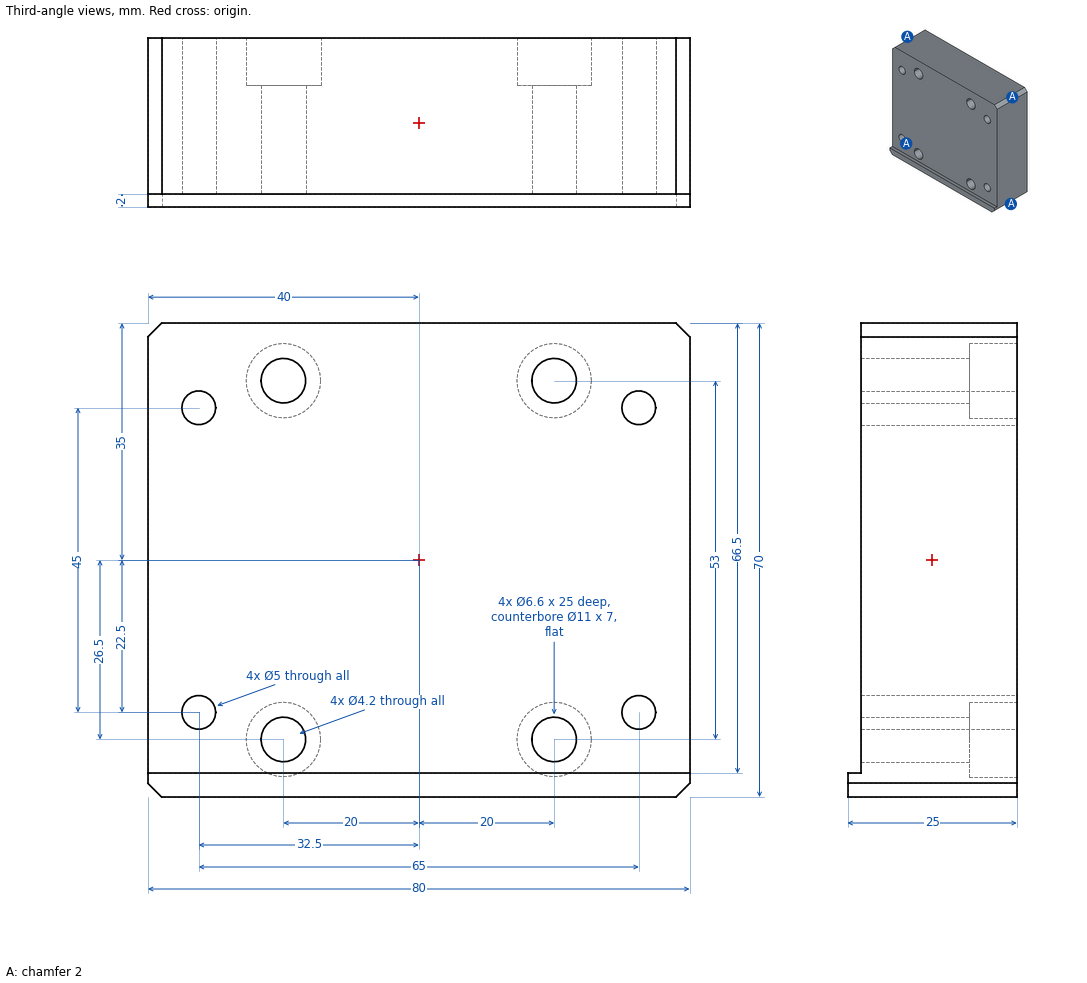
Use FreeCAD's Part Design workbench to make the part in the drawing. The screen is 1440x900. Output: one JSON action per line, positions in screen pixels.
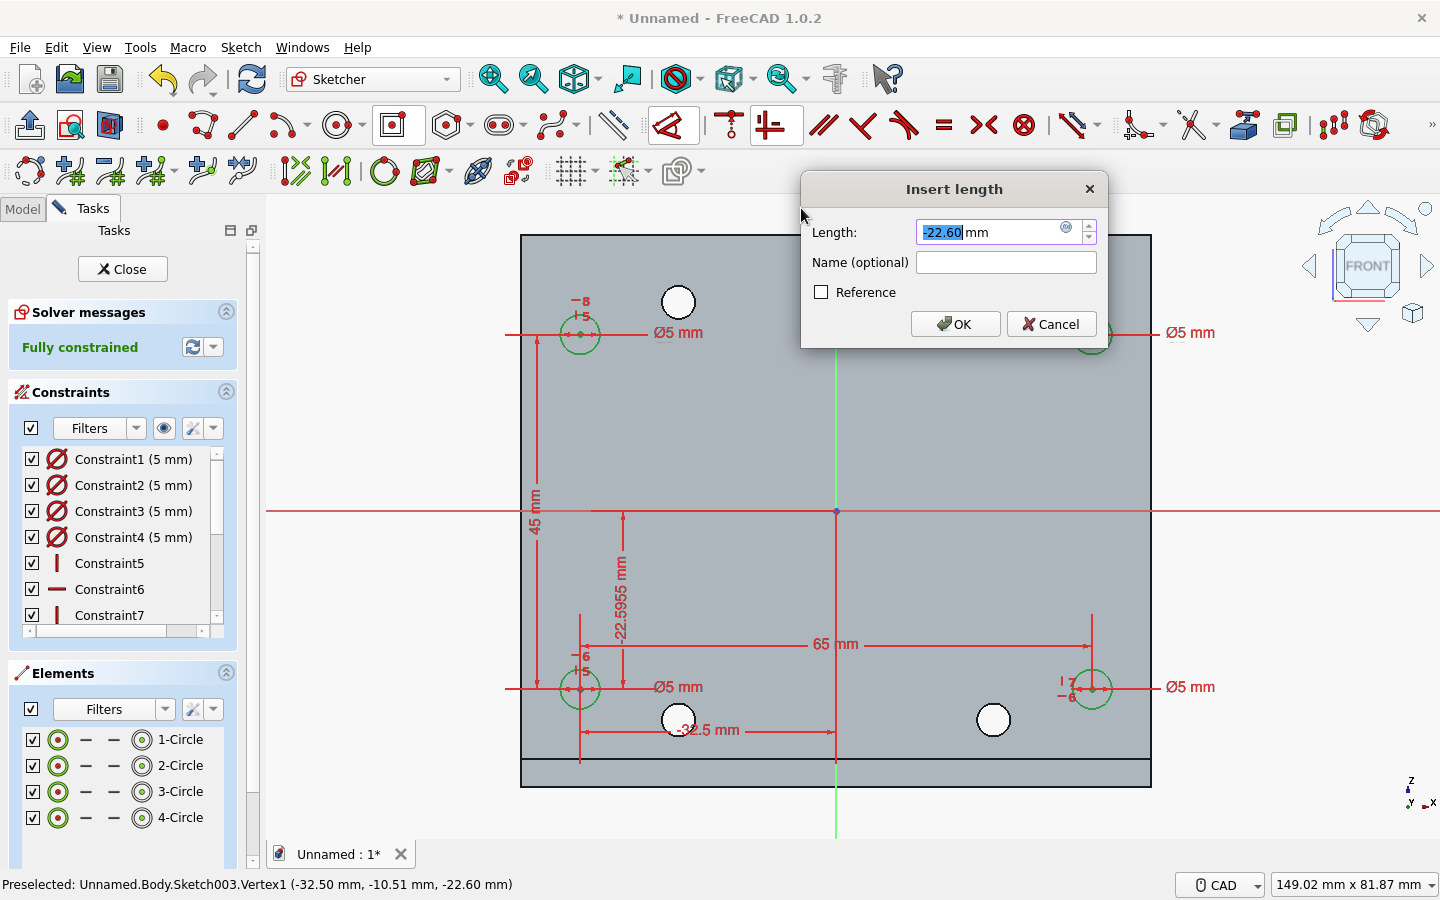
{"action": "type", "text": "-22.5"}
{"action": "key", "text": "Return"}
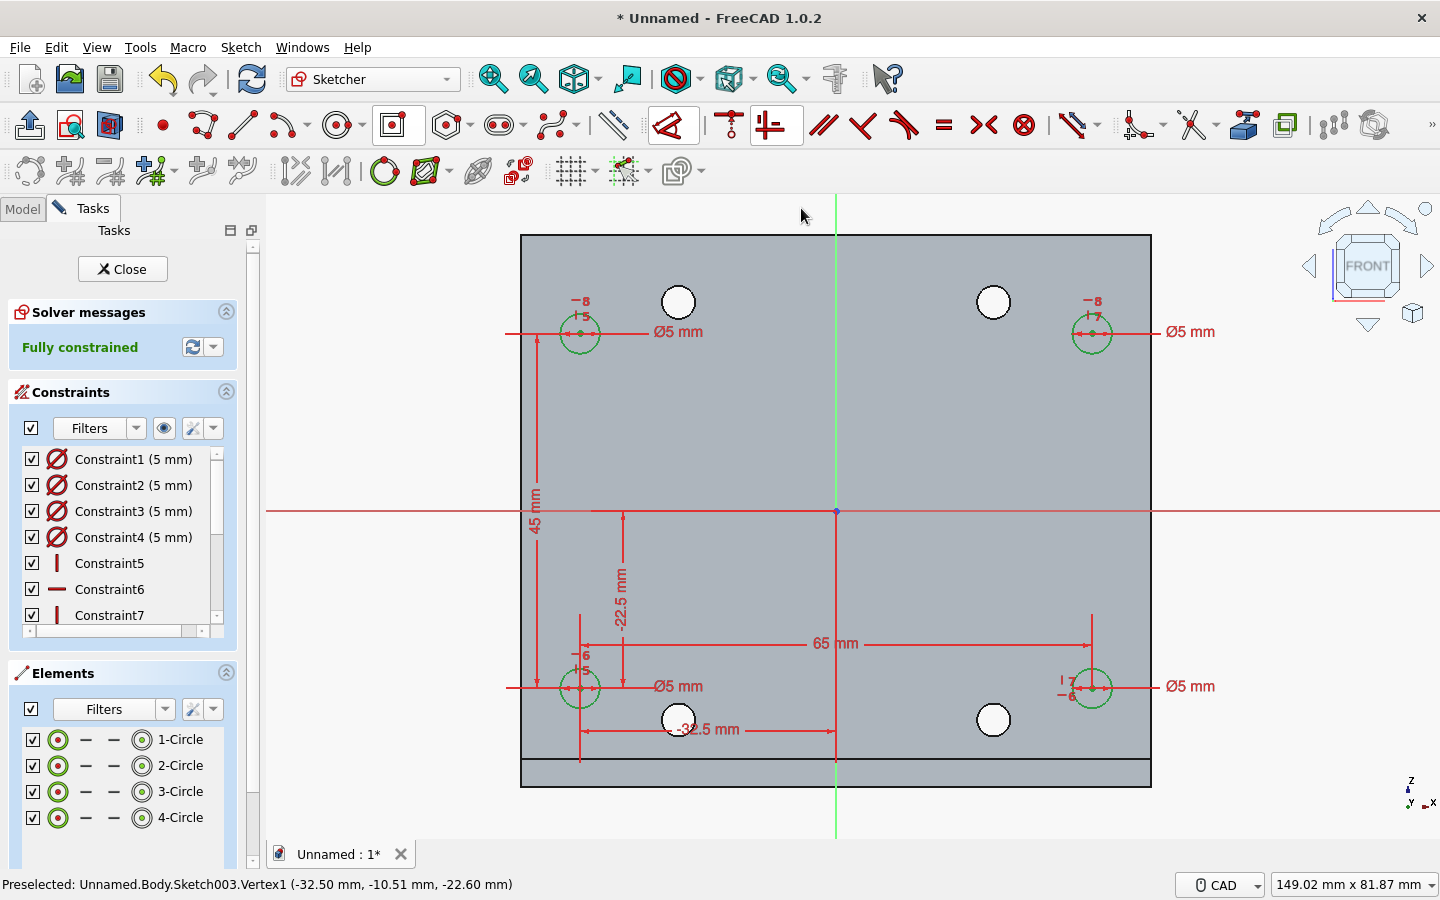
{"action": "left_click", "coordinate": [123, 269]}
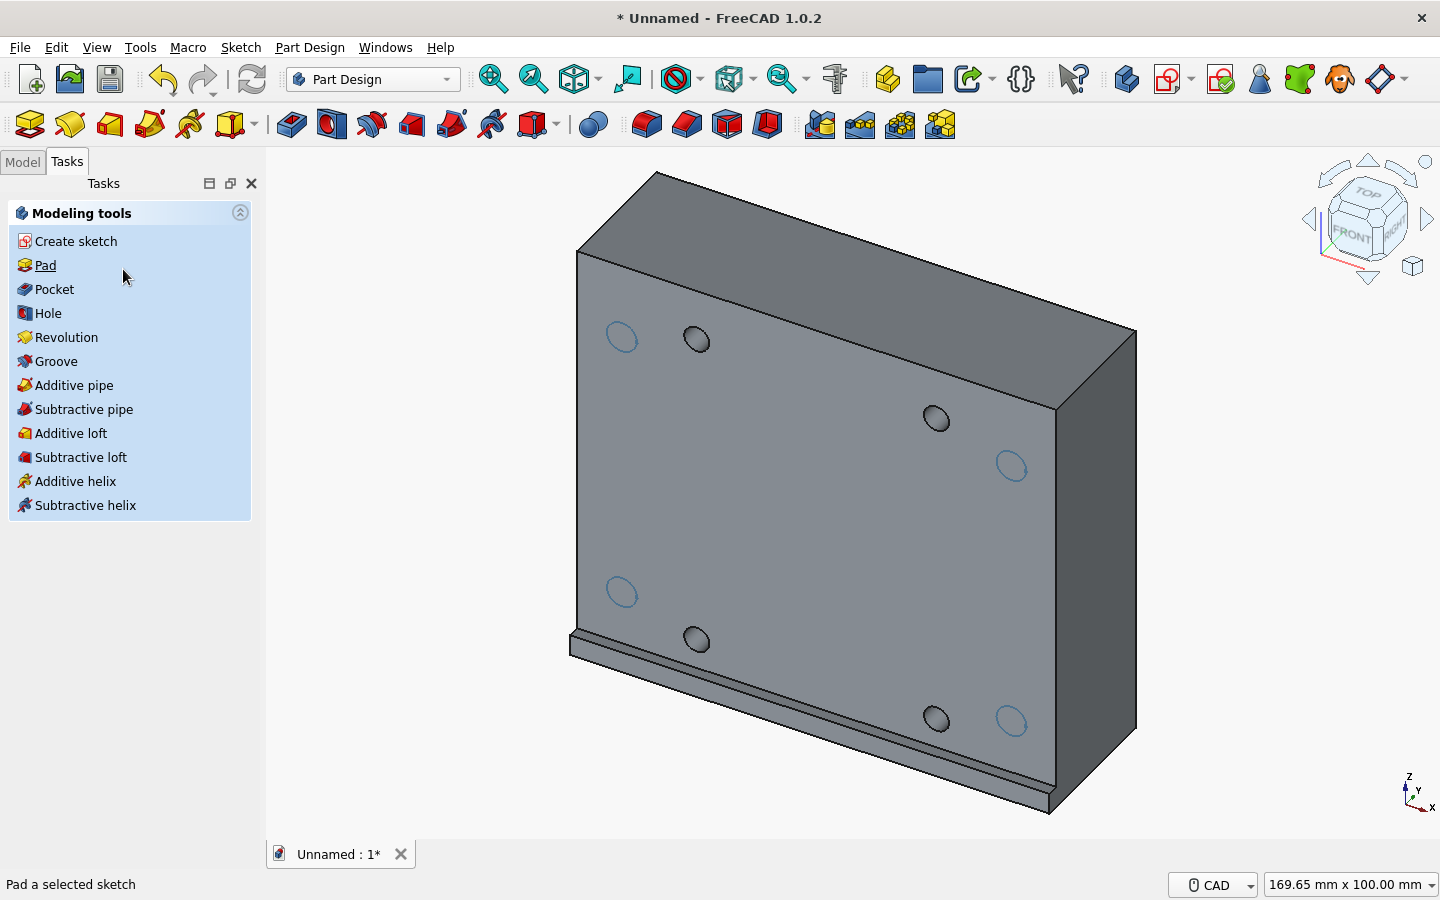
{"action": "left_click", "coordinate": [332, 124]}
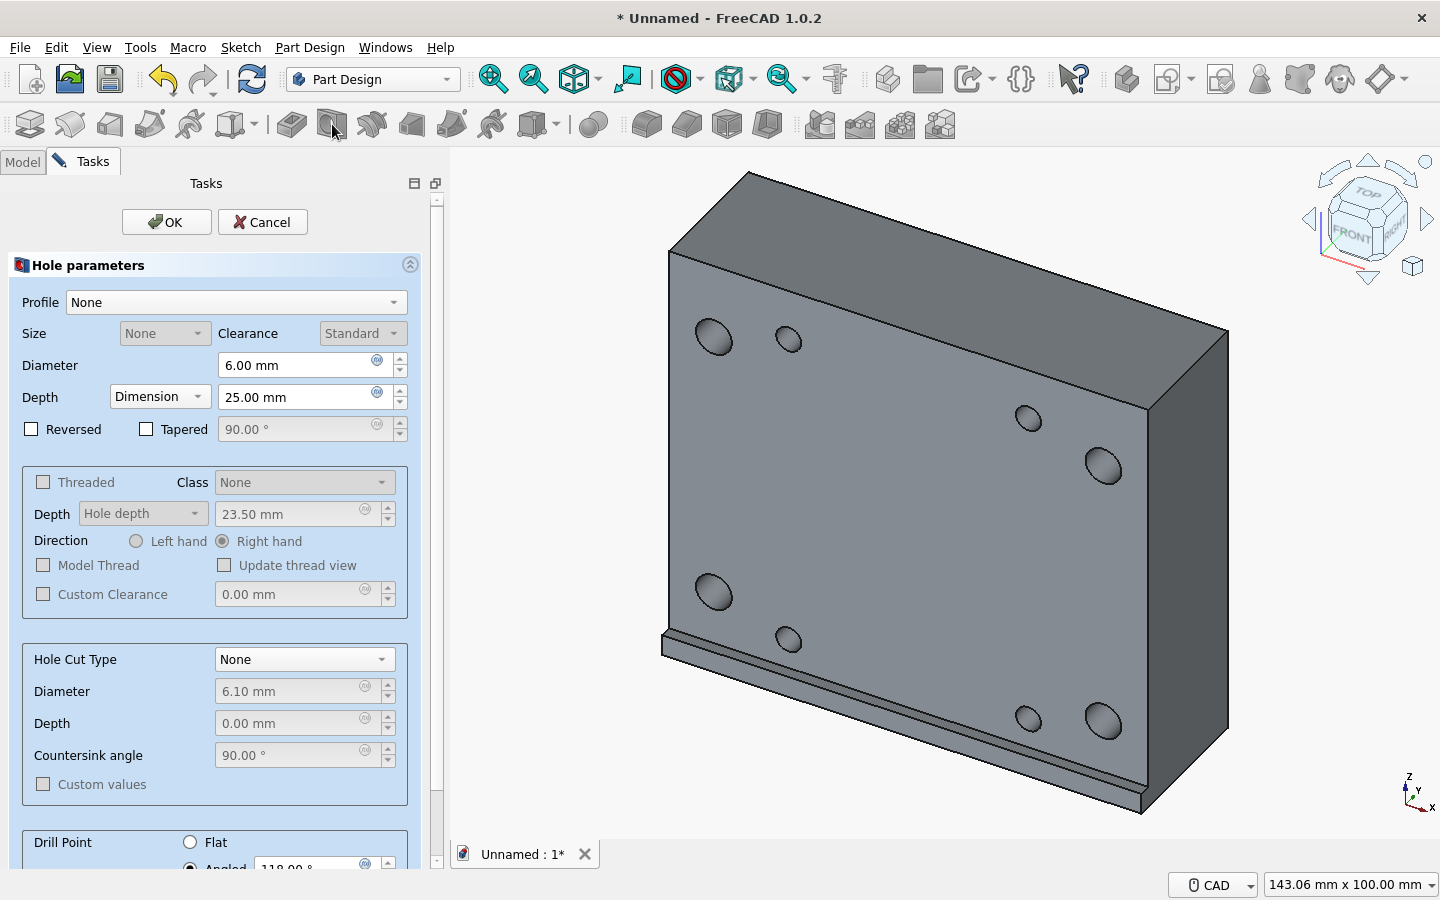
{"action": "triple_click", "coordinate": [305, 365]}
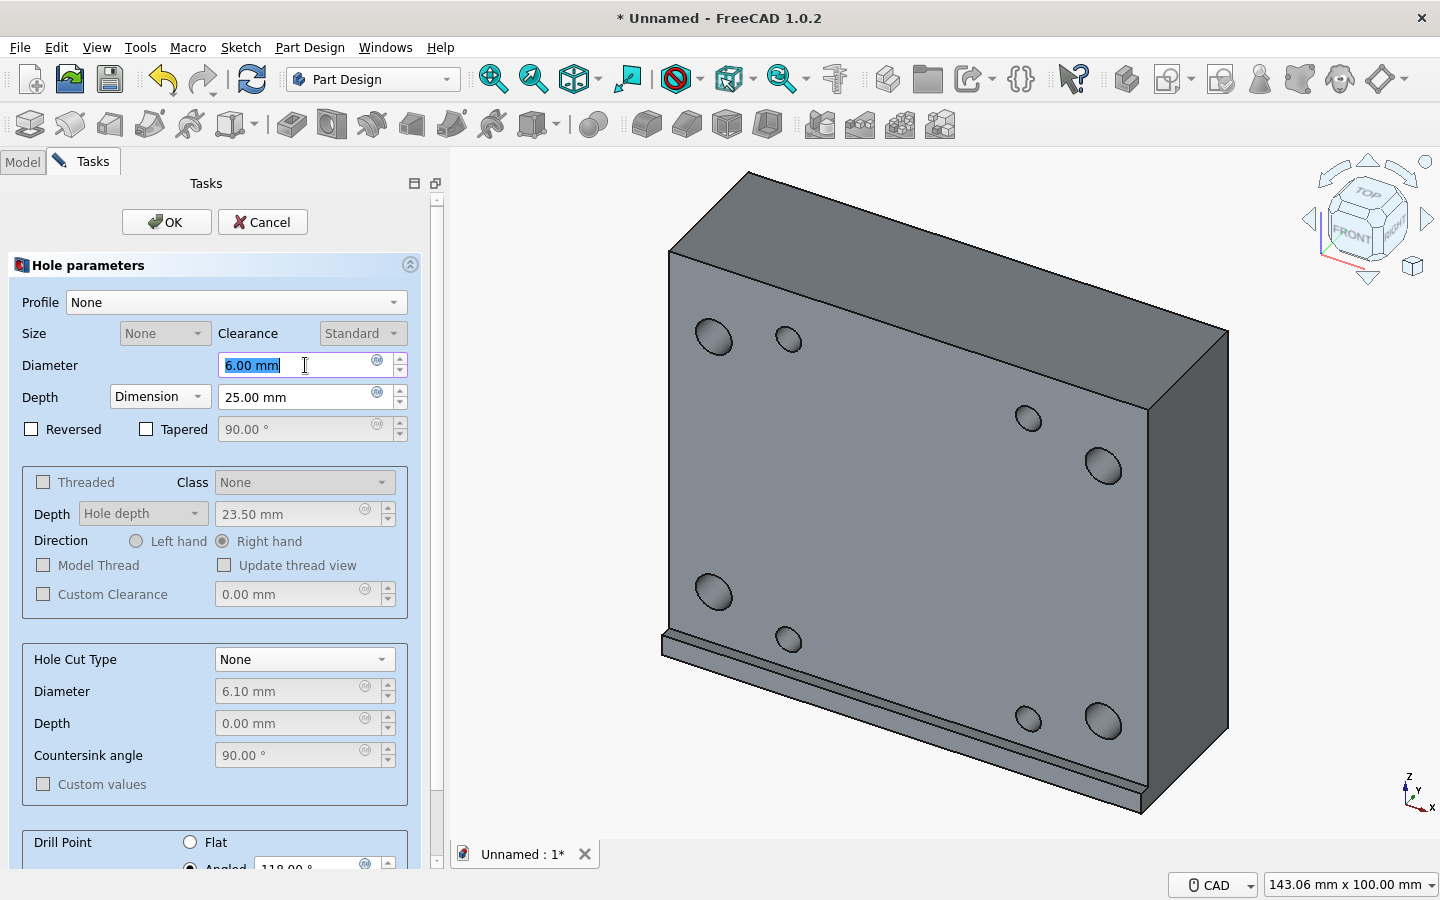
{"action": "type", "text": "5"}
{"action": "key", "text": "Tab"}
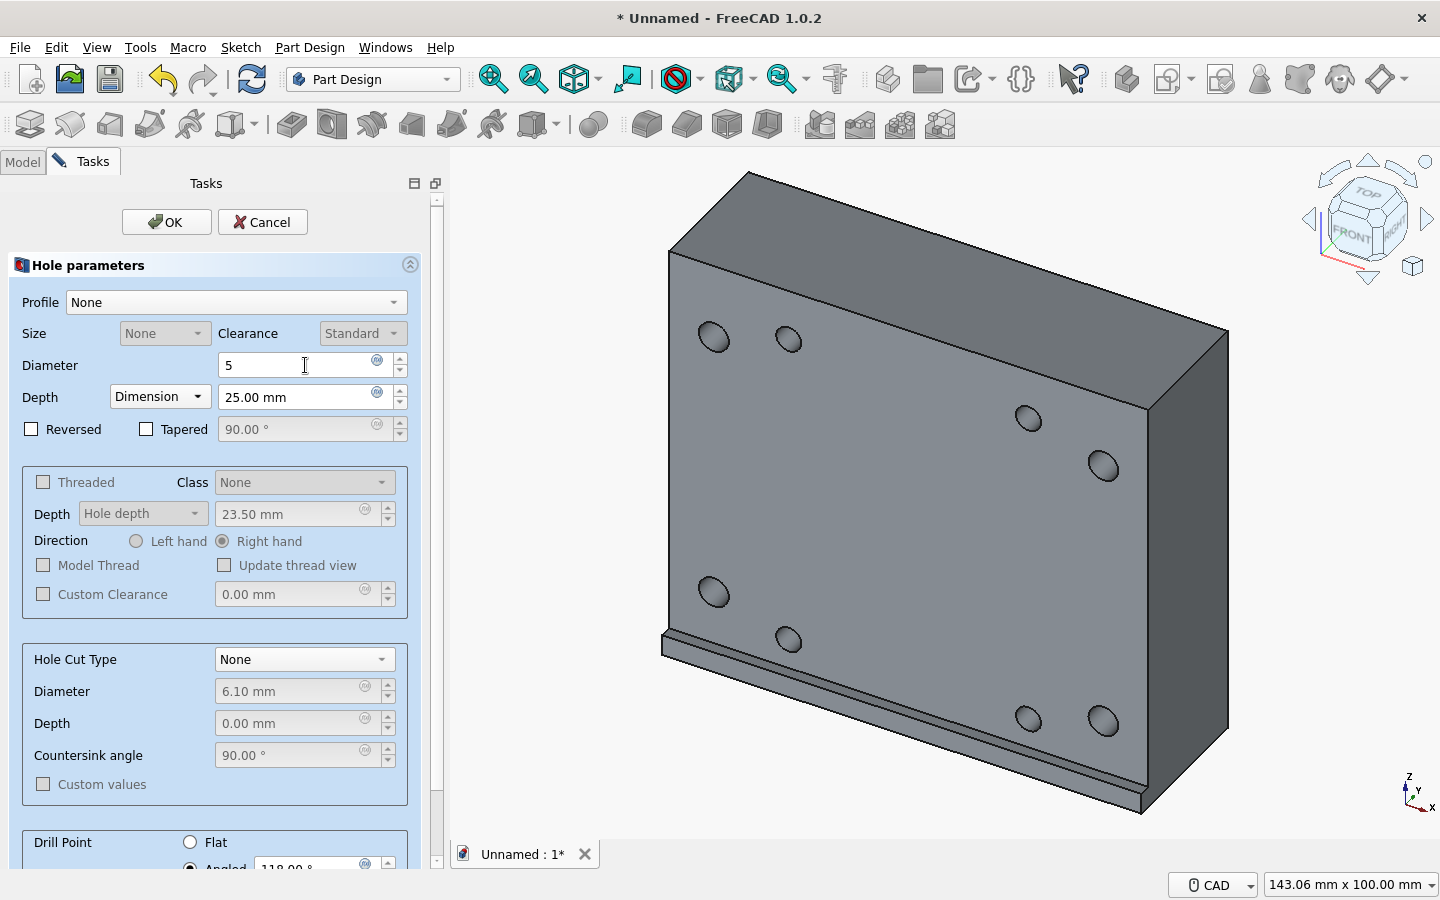
{"action": "left_click", "coordinate": [161, 396]}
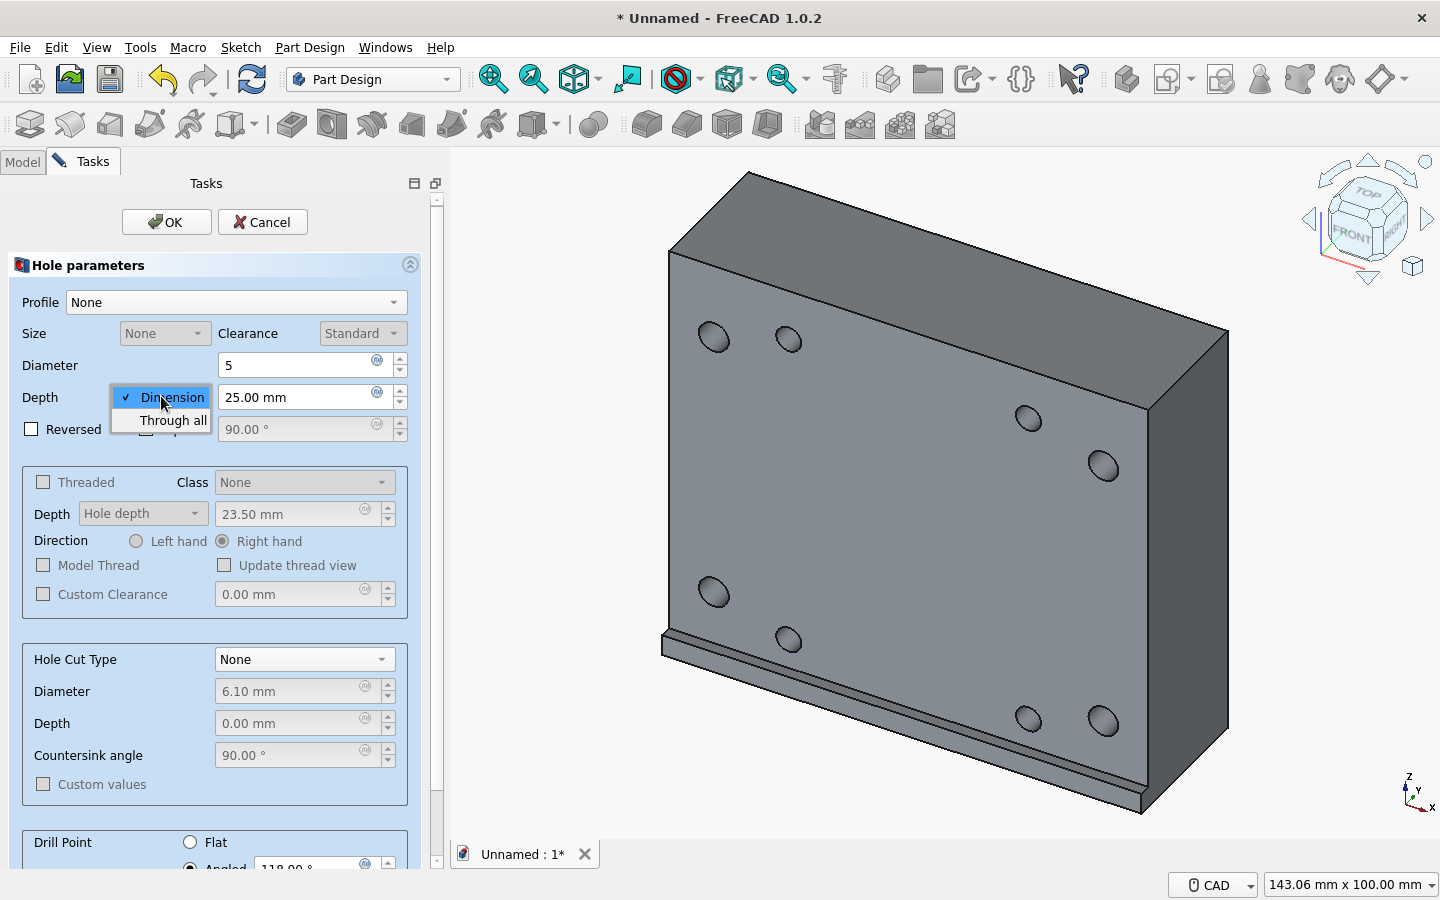
{"action": "left_click", "coordinate": [160, 420]}